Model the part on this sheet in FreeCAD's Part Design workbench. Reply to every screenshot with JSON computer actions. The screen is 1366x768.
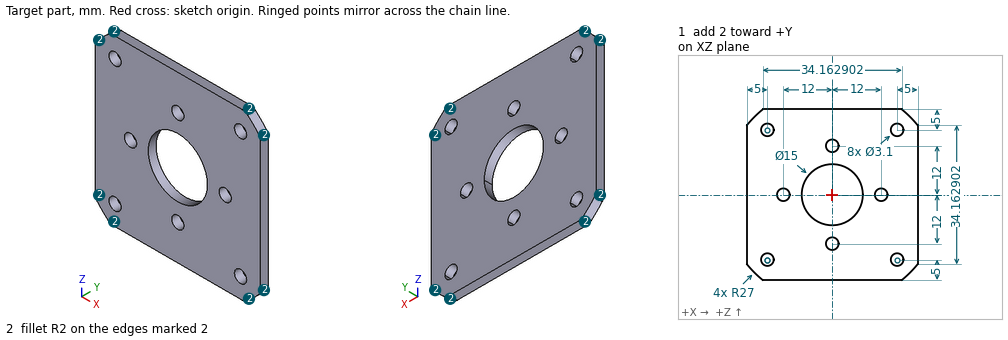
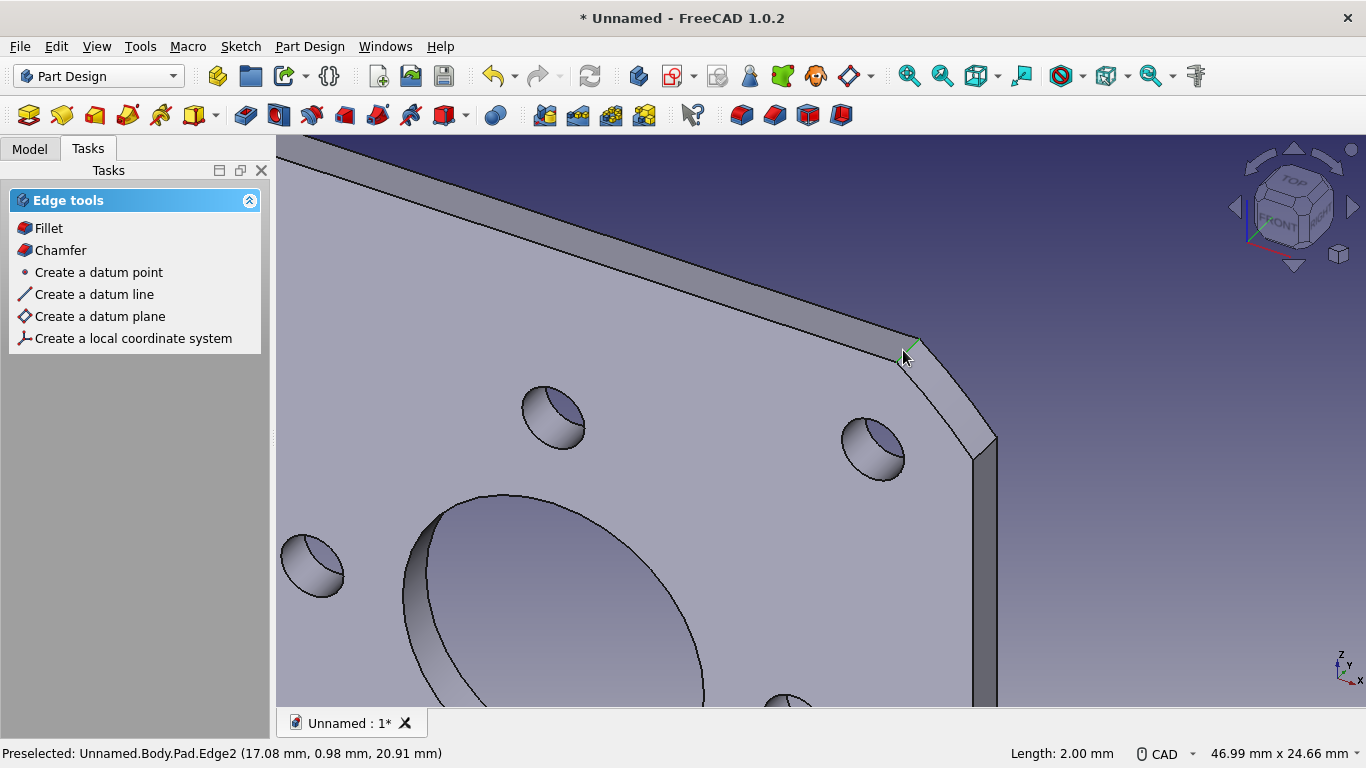
{"action": "left_click", "coordinate": [910, 76]}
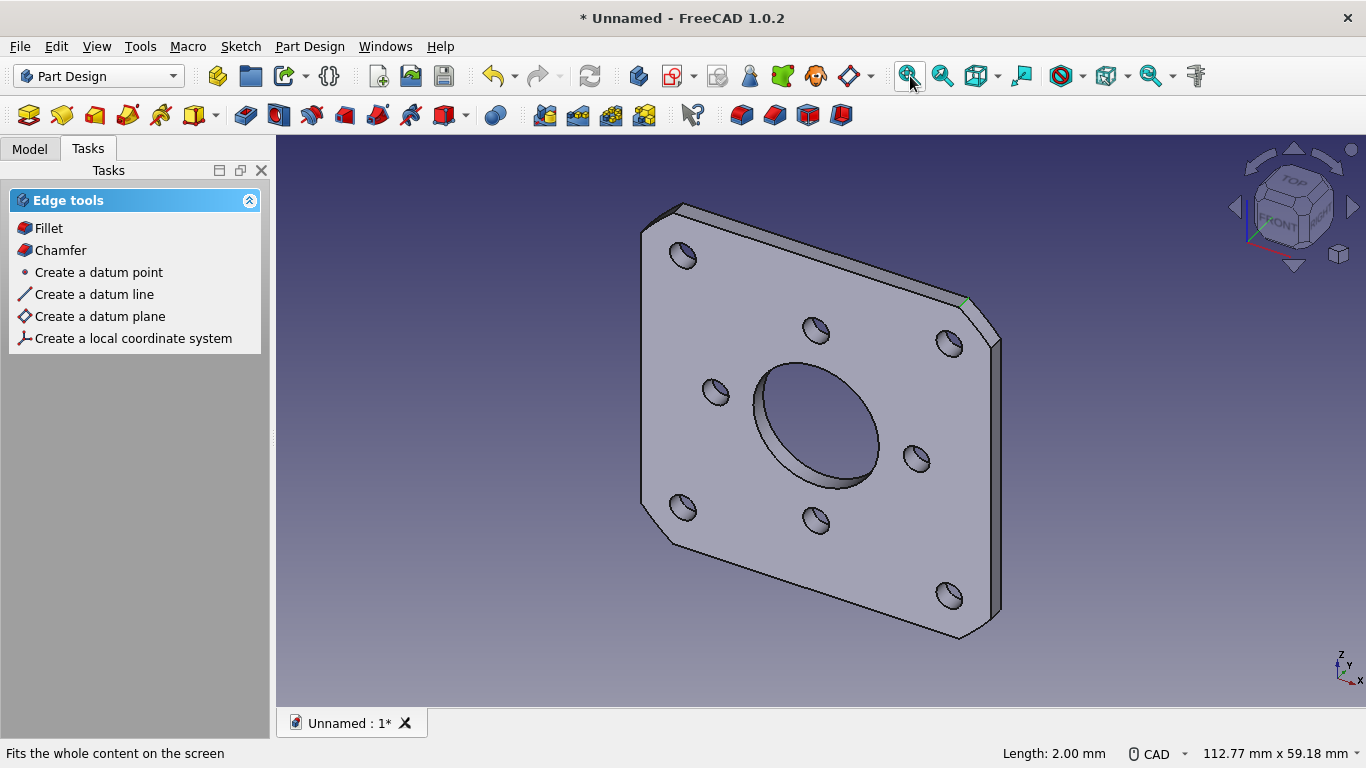
{"action": "key", "text": "0"}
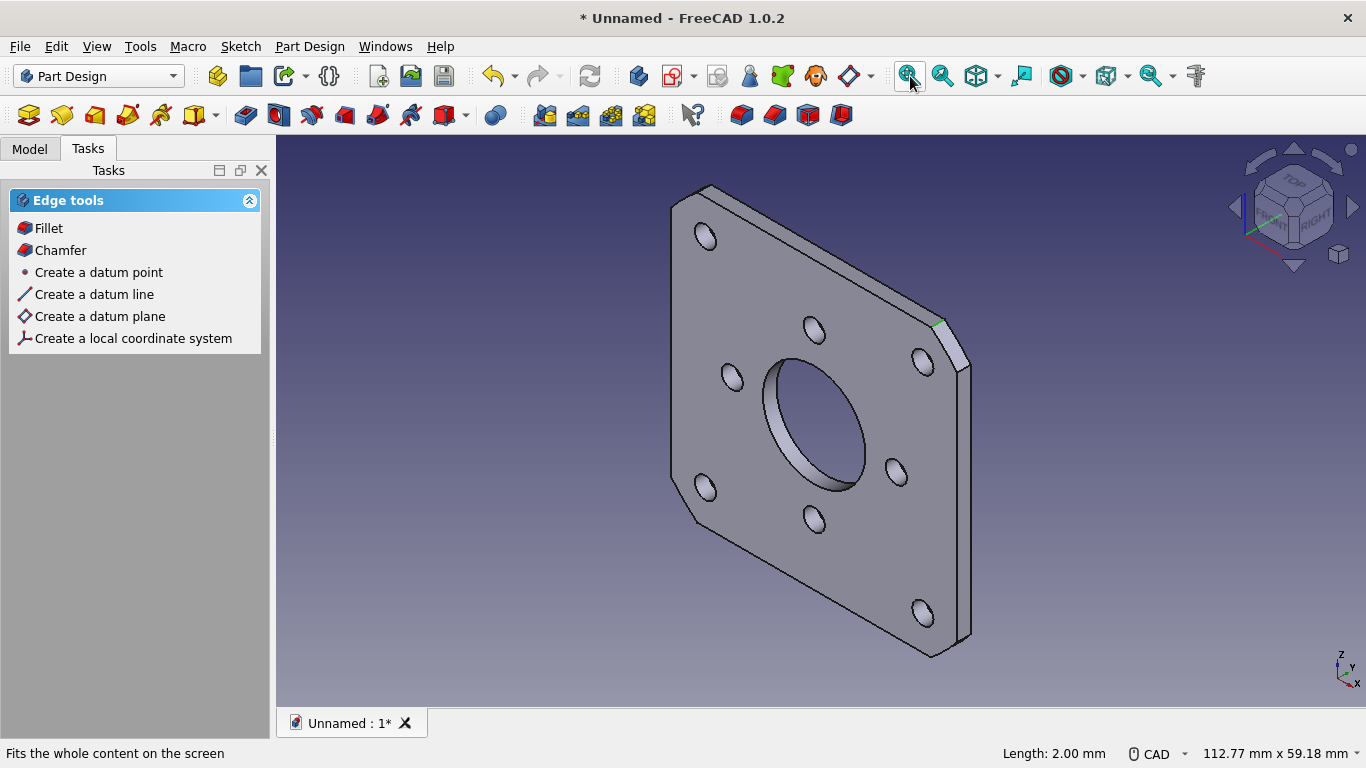
{"action": "scroll", "coordinate": [704, 188], "scroll_direction": "up", "scroll_amount": 4}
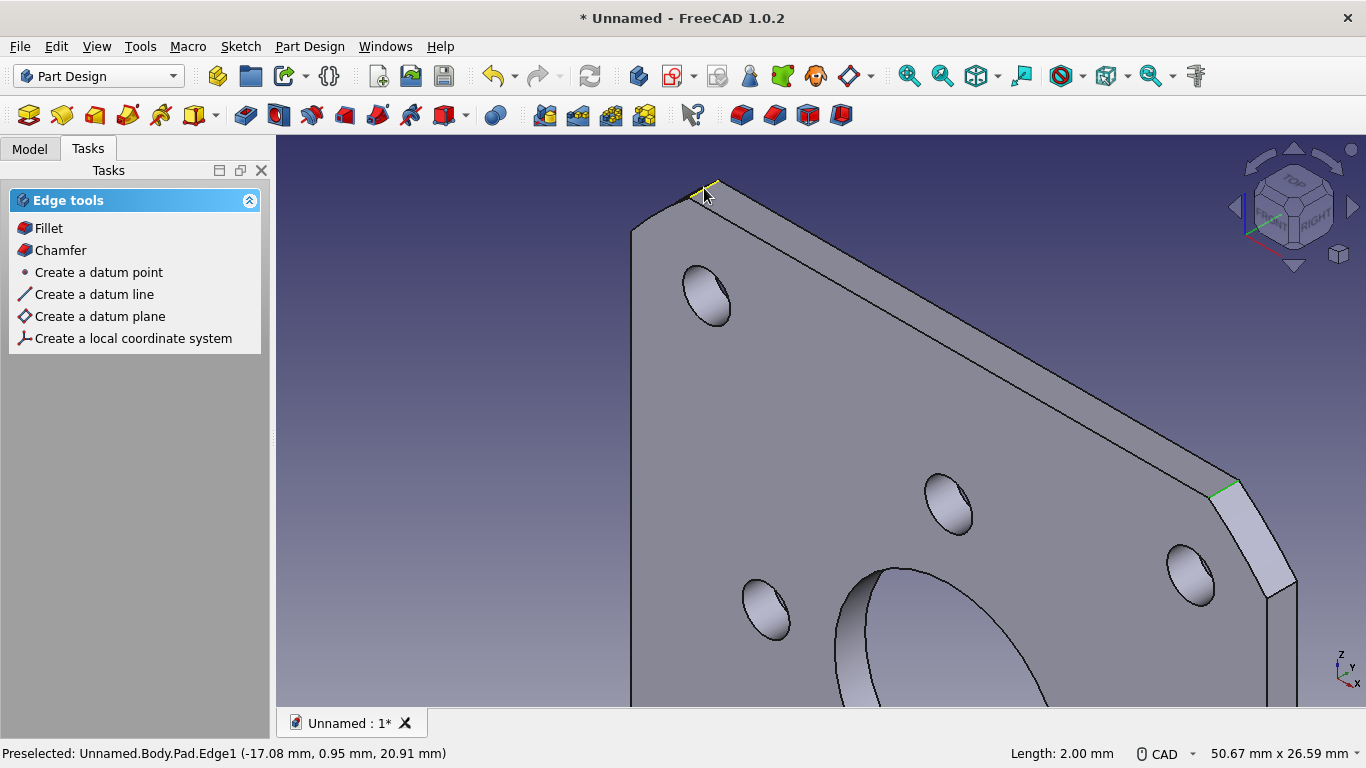
{"action": "left_click", "coordinate": [910, 76]}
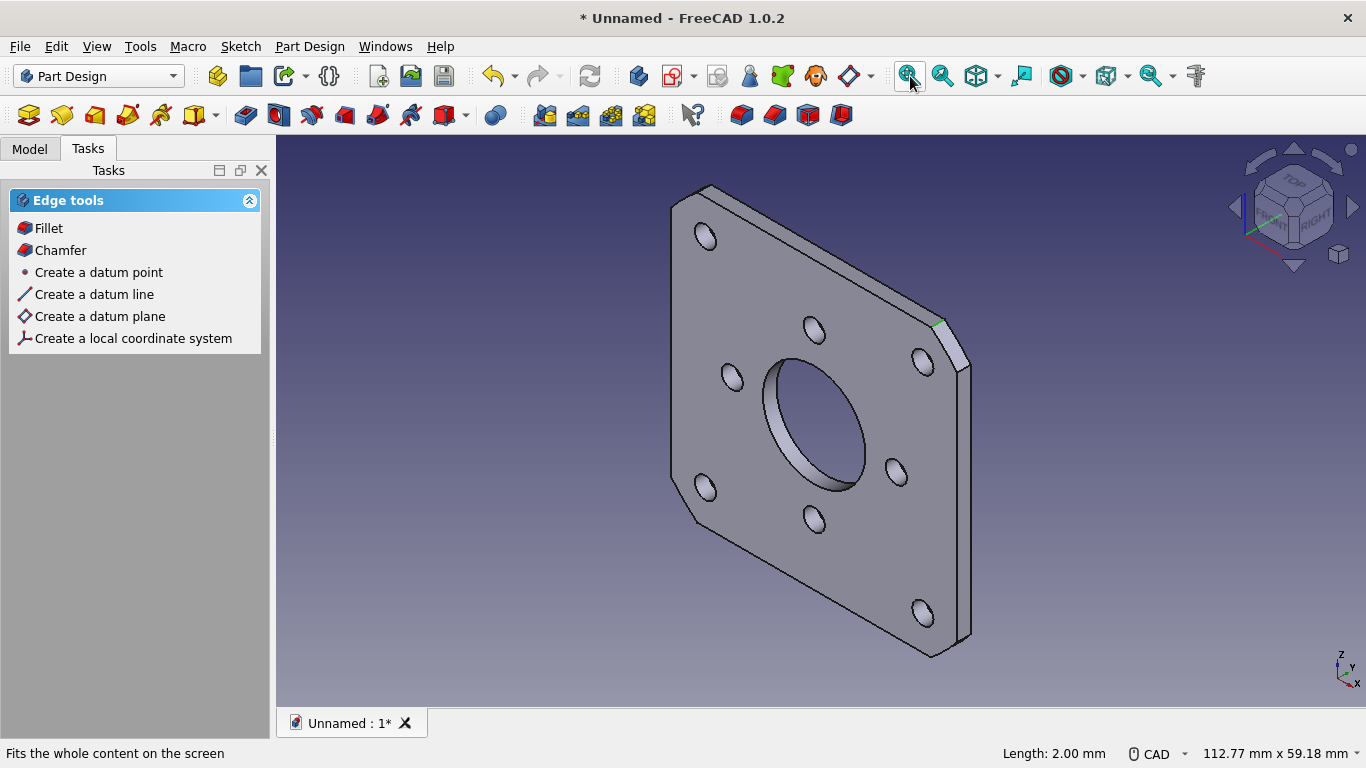
{"action": "key", "text": "2"}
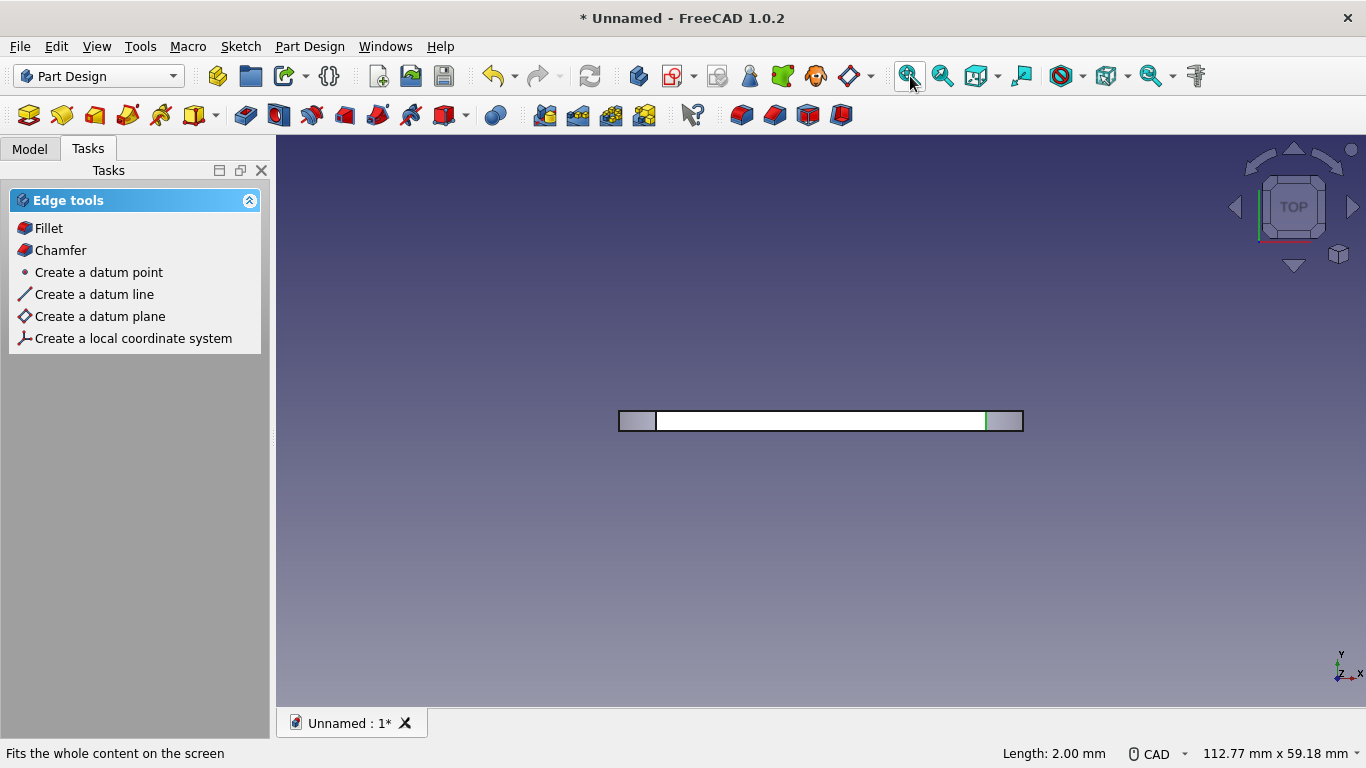
{"action": "left_click", "coordinate": [910, 76]}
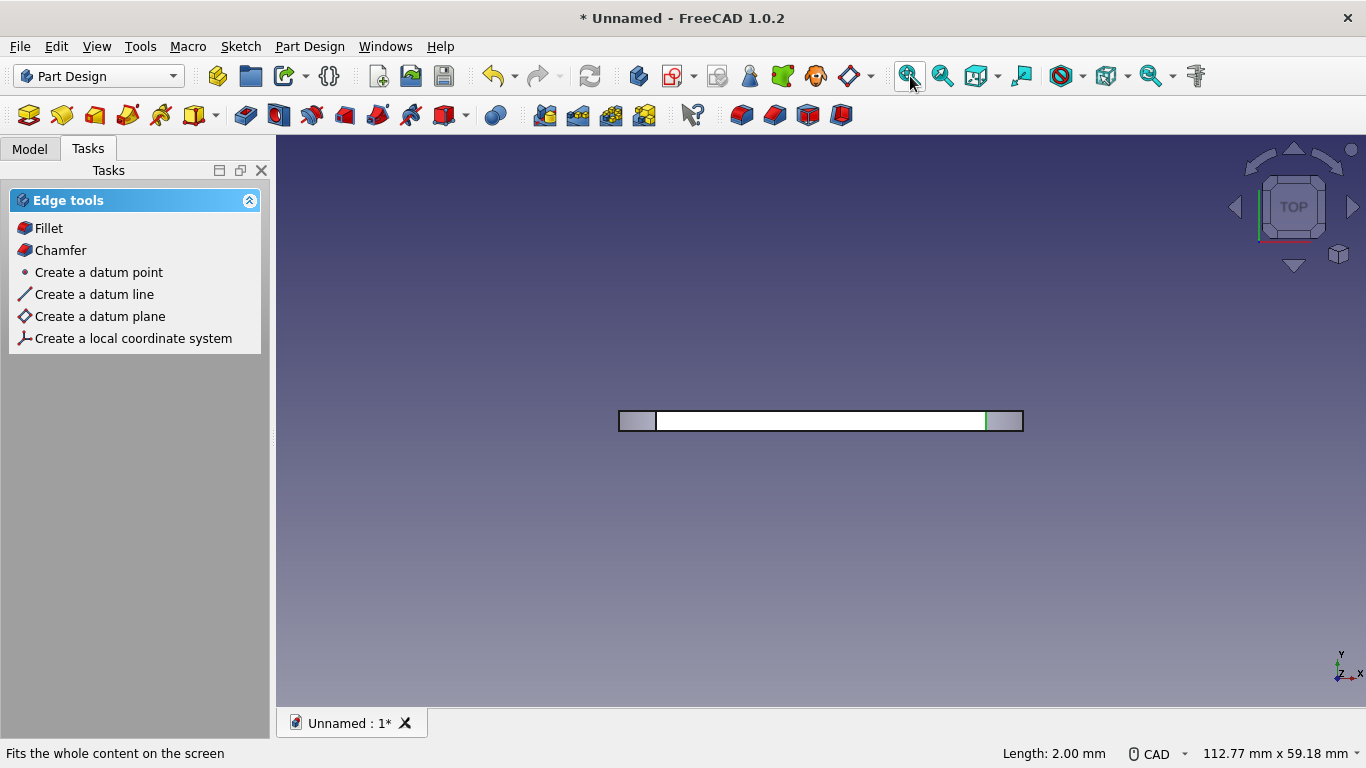
{"action": "left_click", "coordinate": [656, 420], "text": "ctrl"}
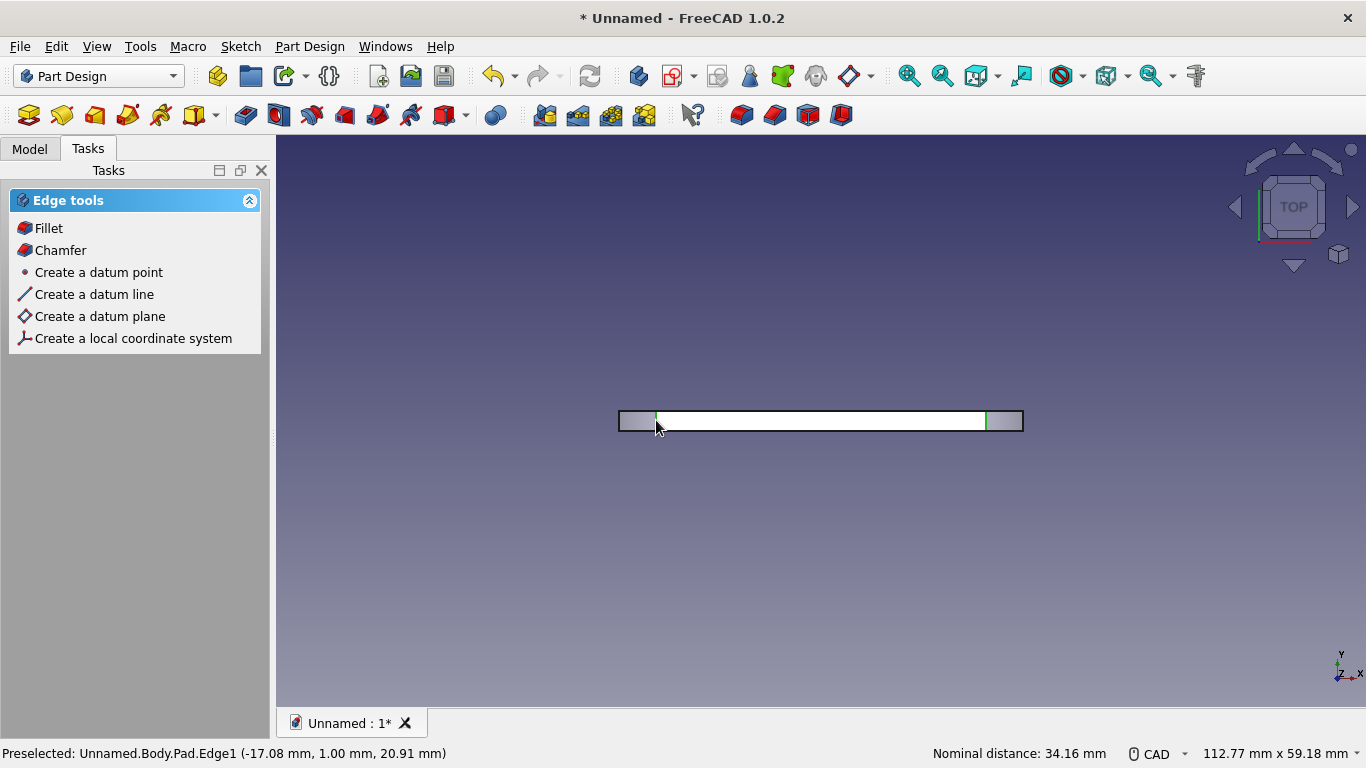
{"action": "scroll", "coordinate": [619, 420], "scroll_direction": "up", "scroll_amount": 4}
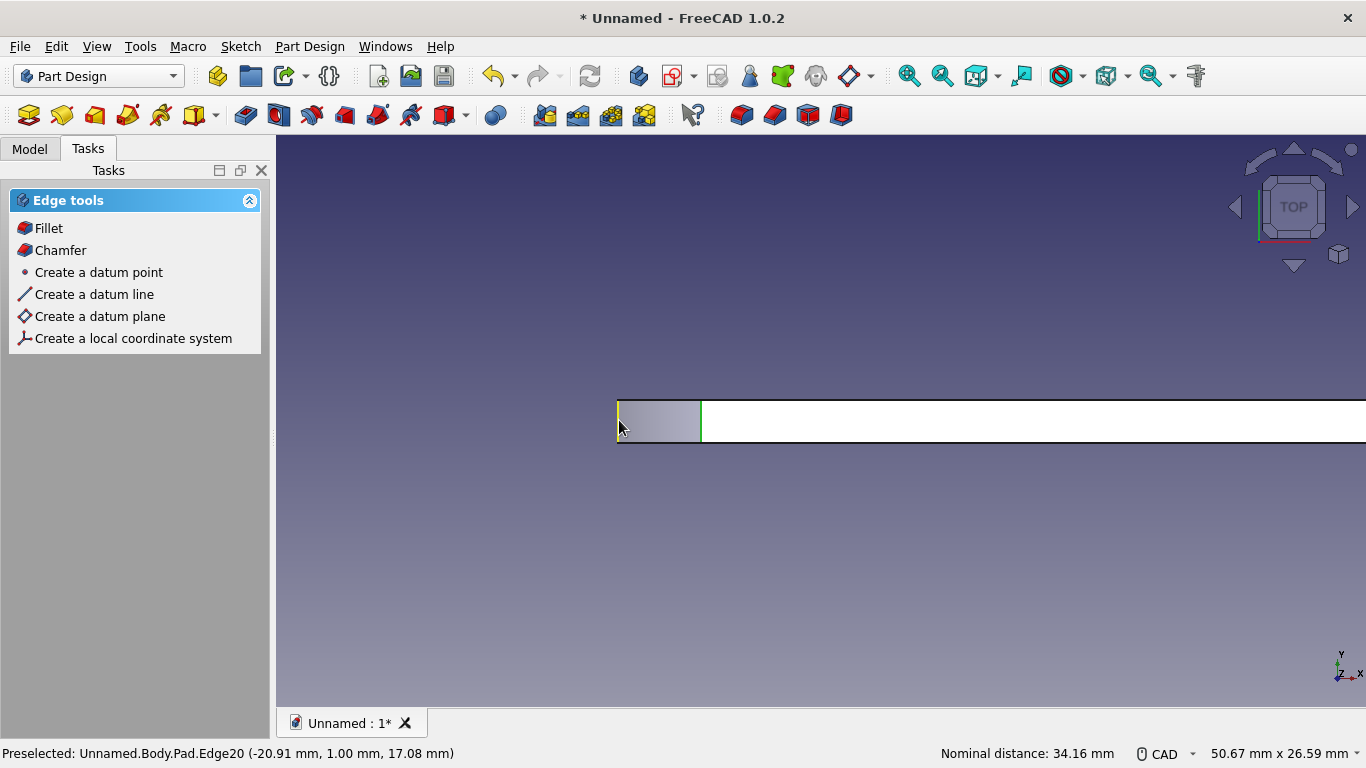
{"action": "left_click", "coordinate": [910, 76]}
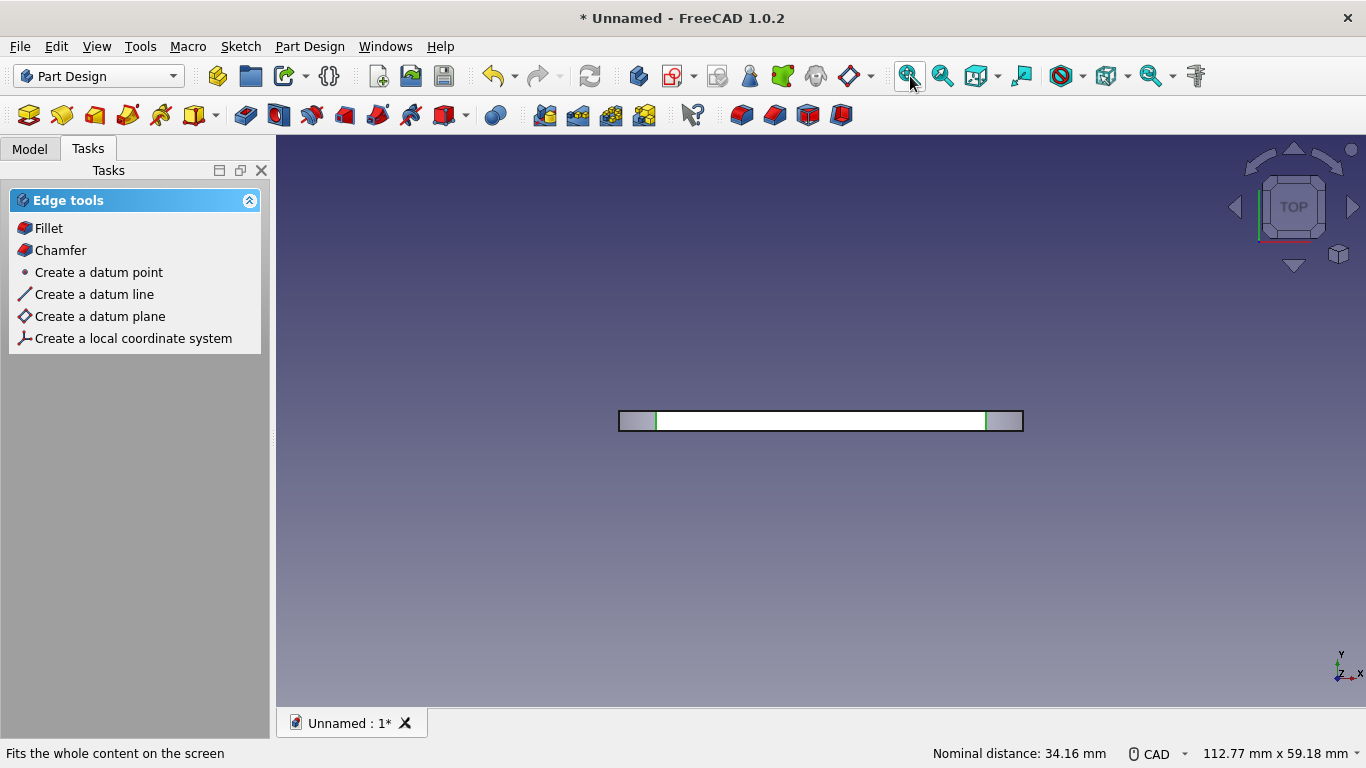
{"action": "key", "text": "1"}